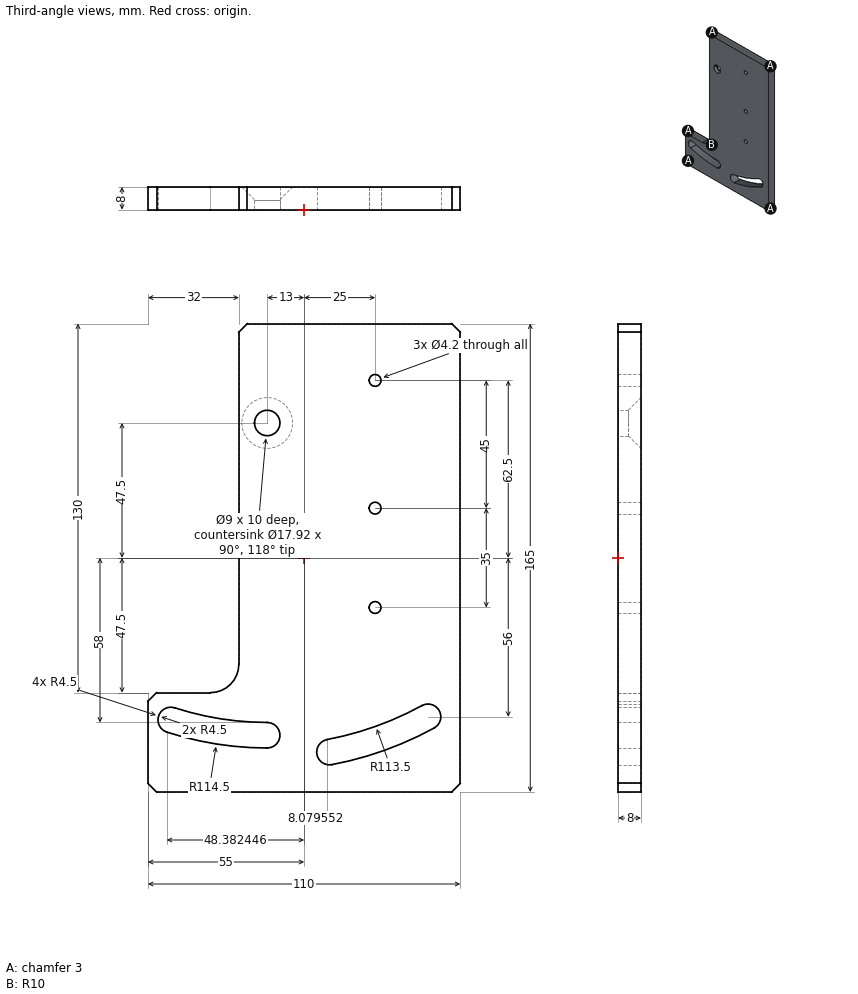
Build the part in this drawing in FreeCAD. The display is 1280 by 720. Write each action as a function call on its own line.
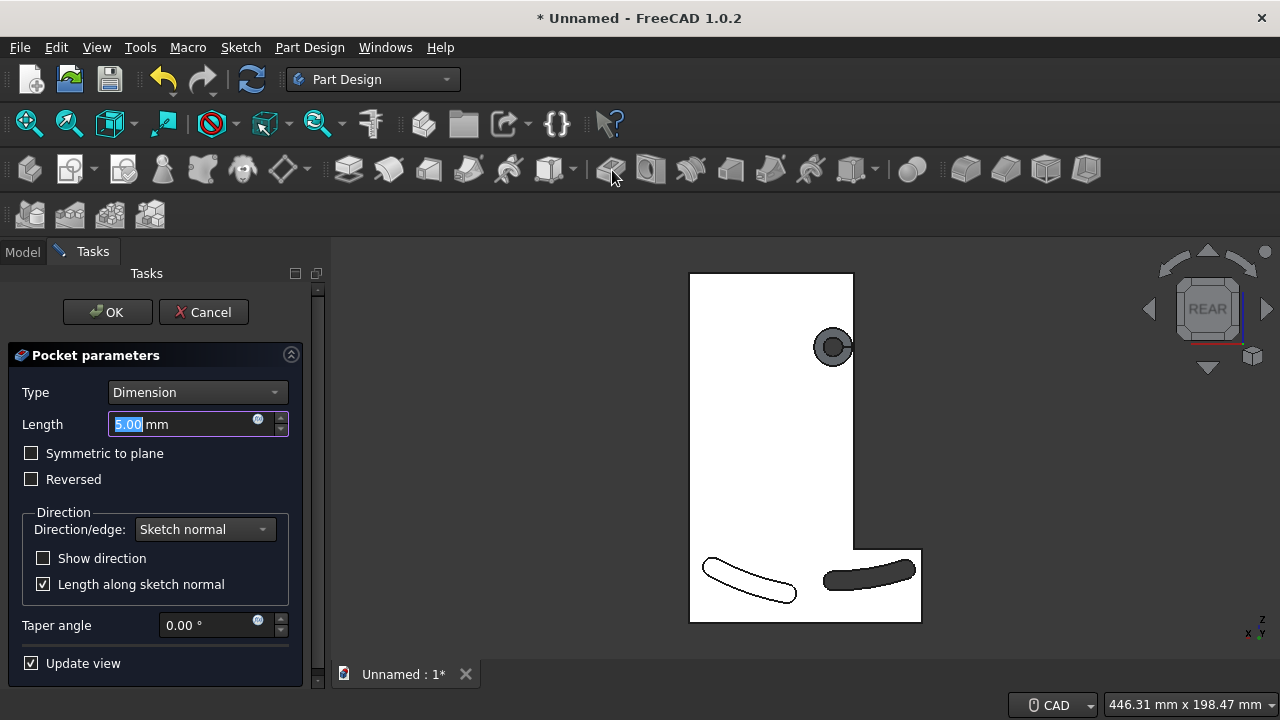
text(8)
key(Tab)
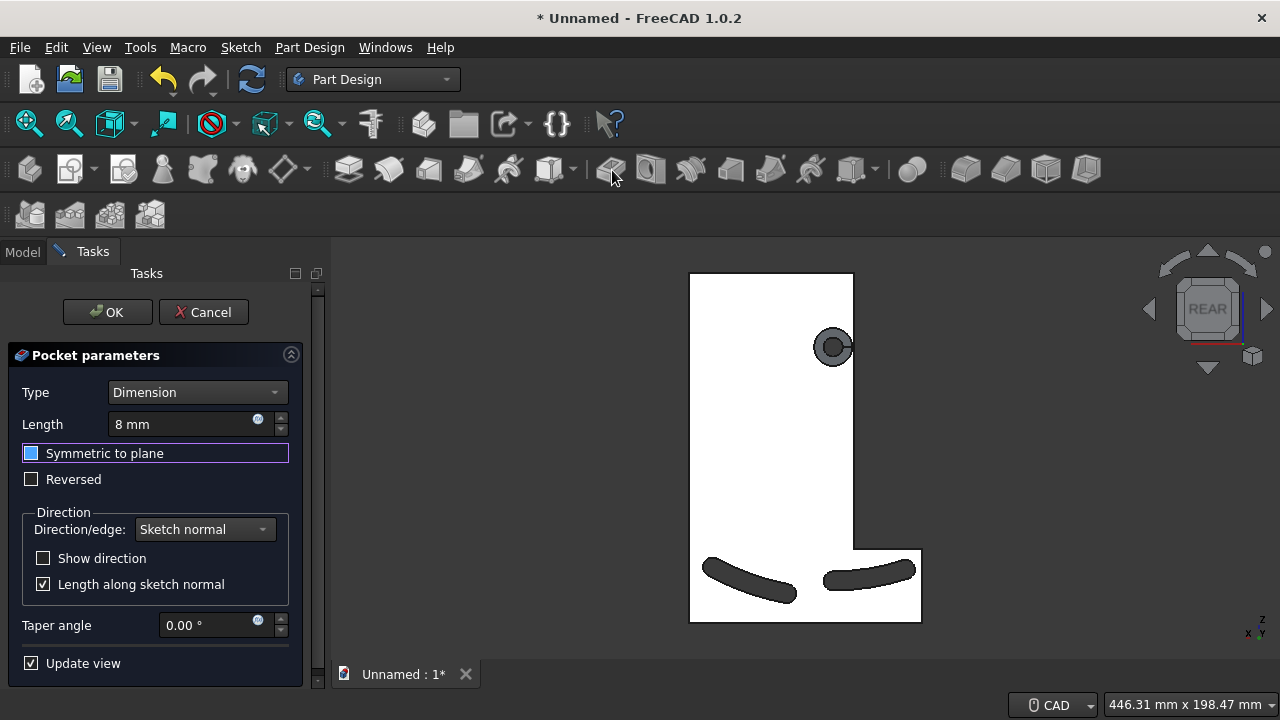
click(108, 312)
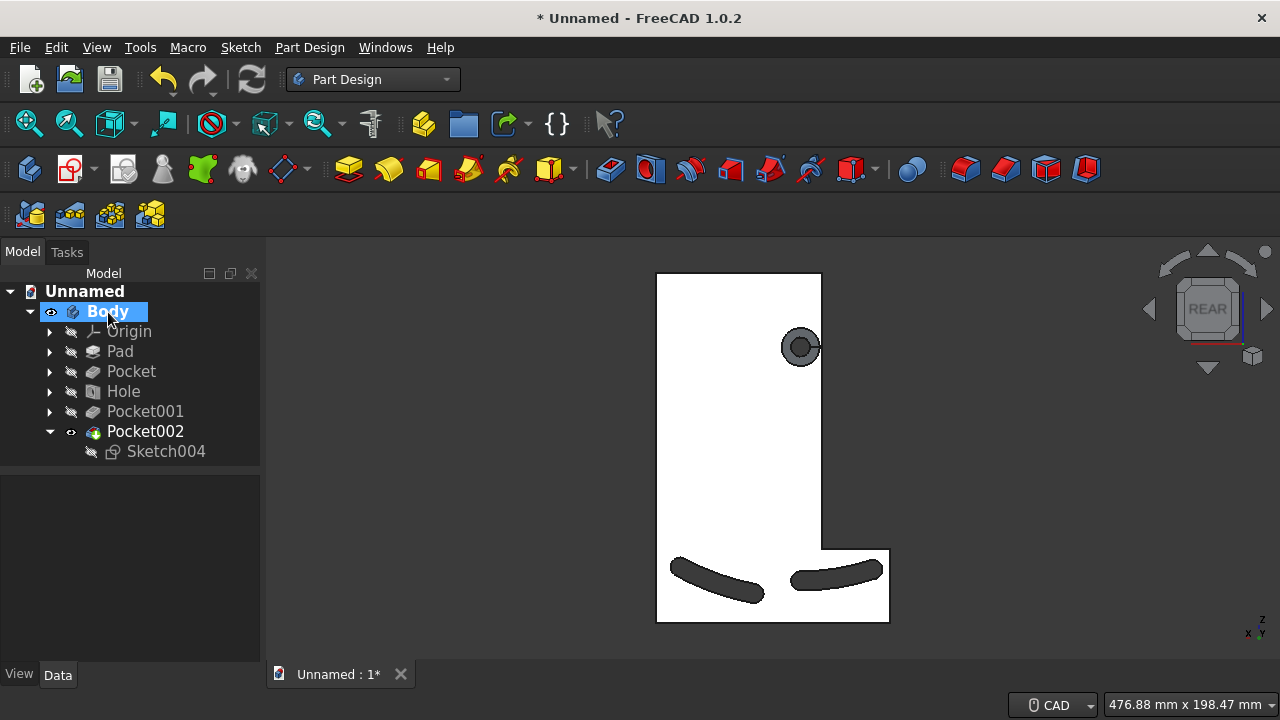
scroll(890, 548, up, 5)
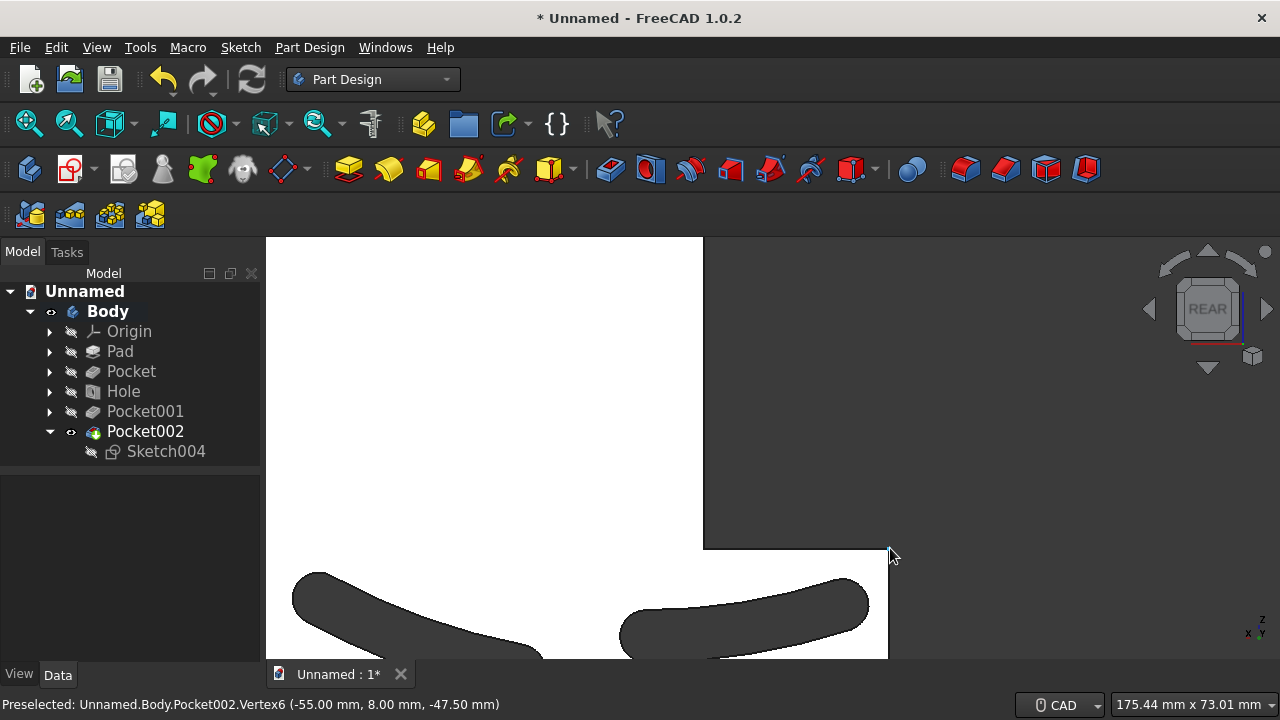
click(30, 124)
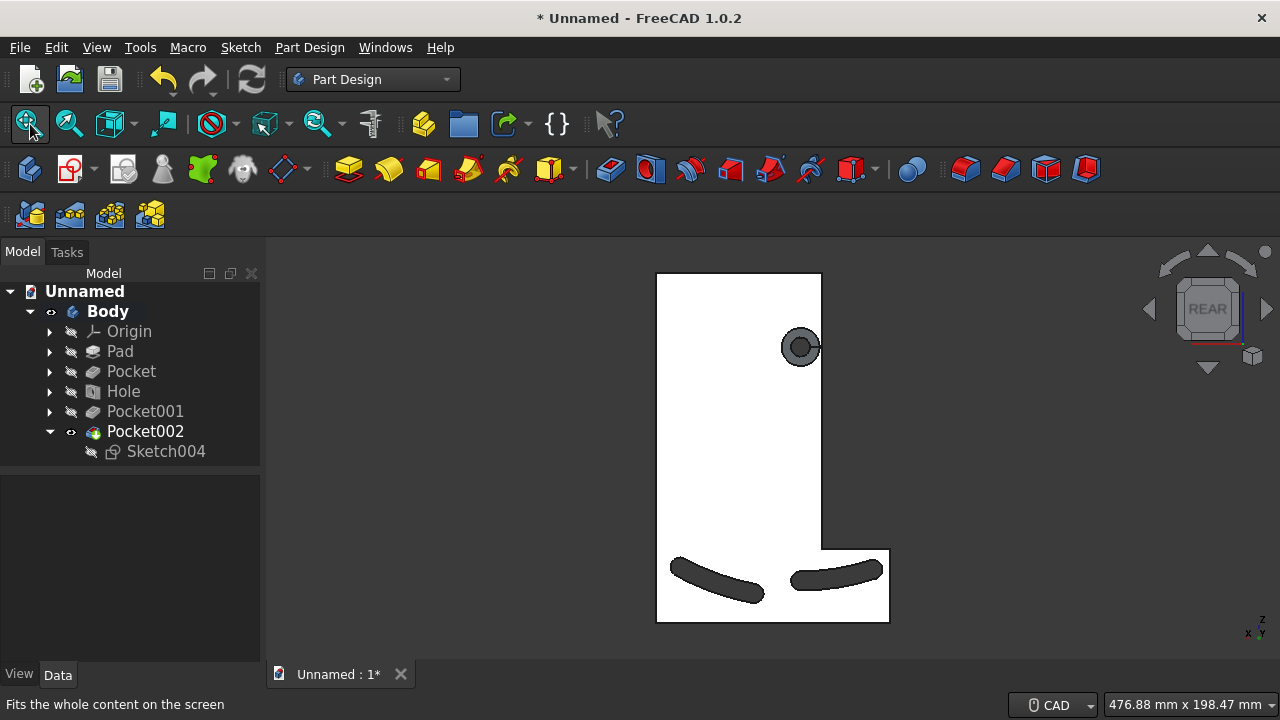
key(0)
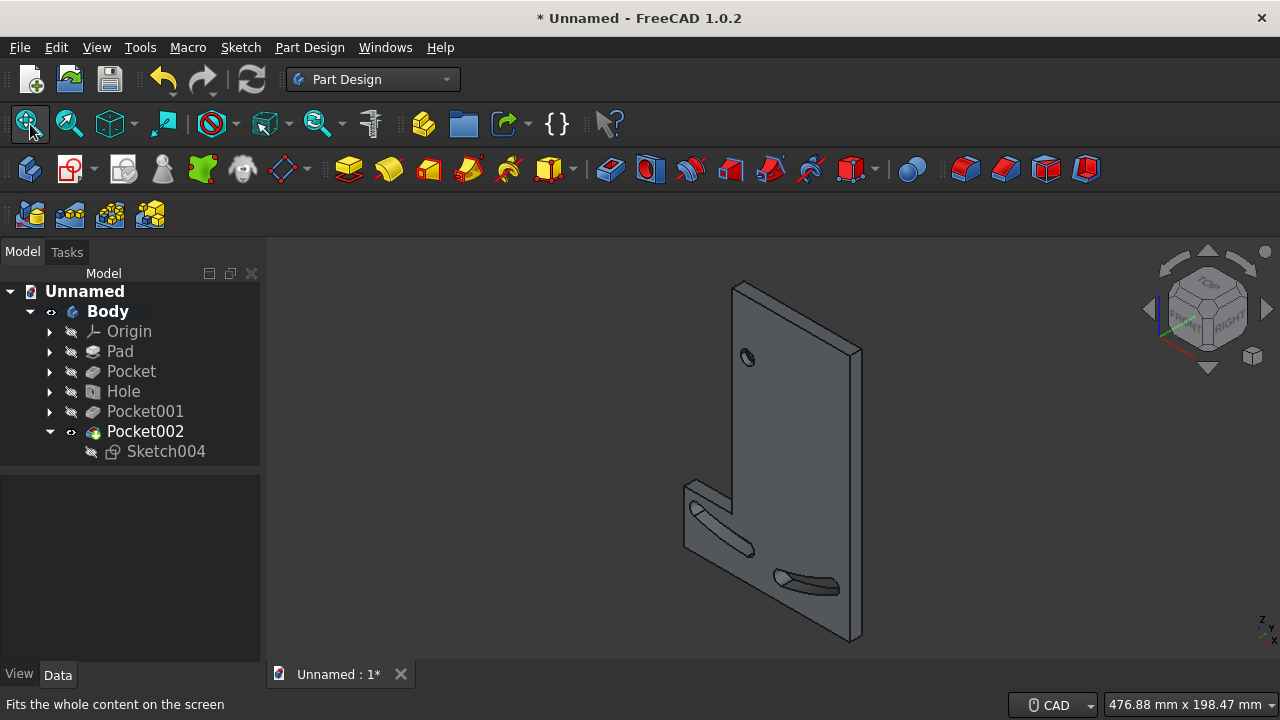
click(856, 352)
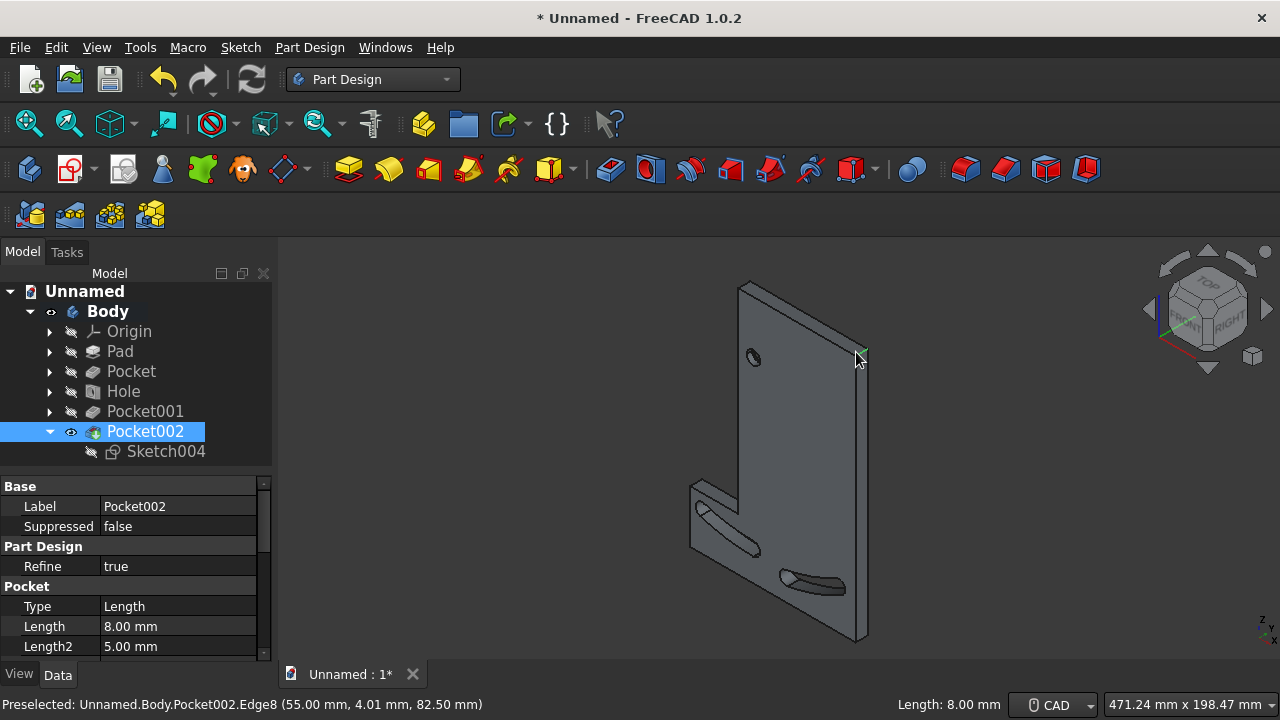
scroll(696, 482, up, 5)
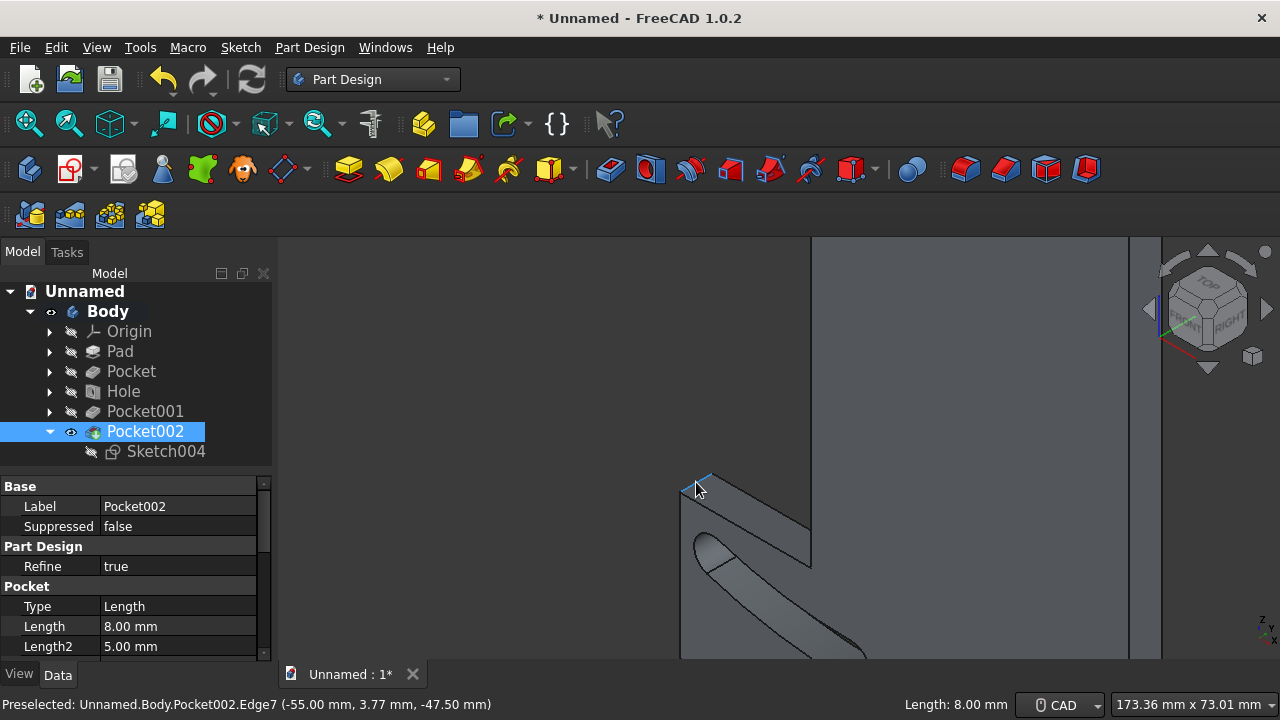
click(30, 124)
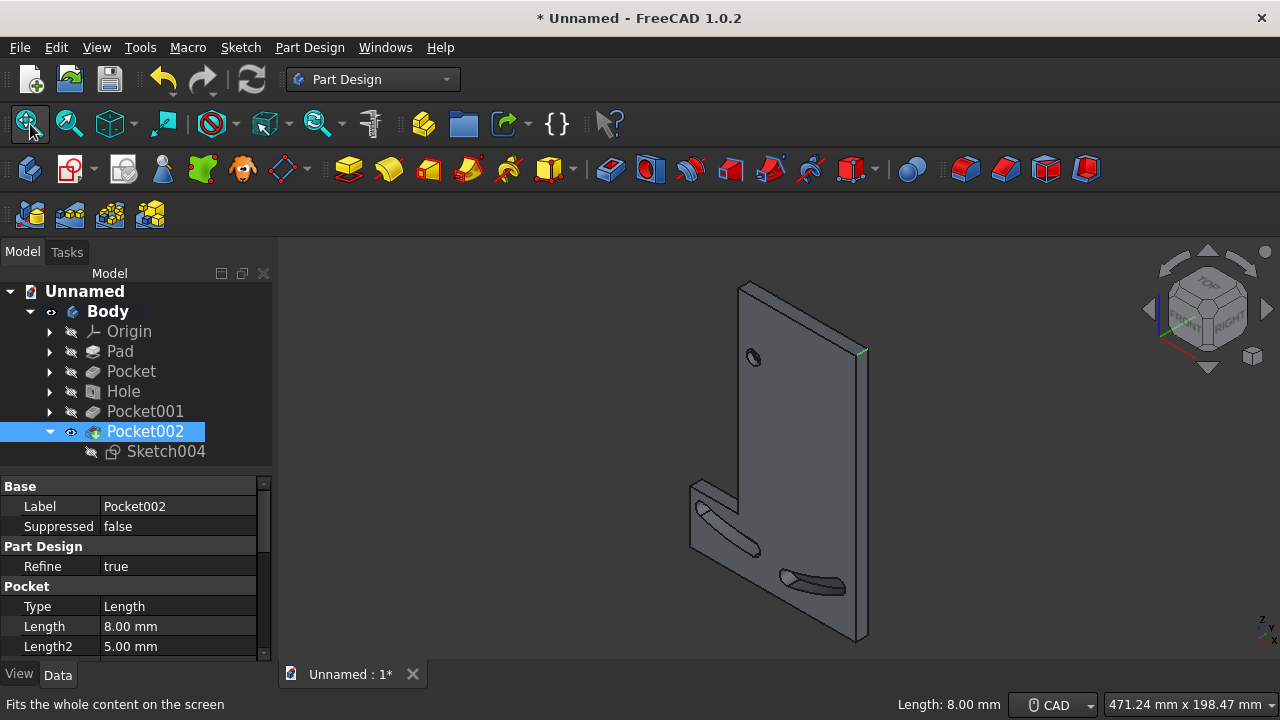
key(2)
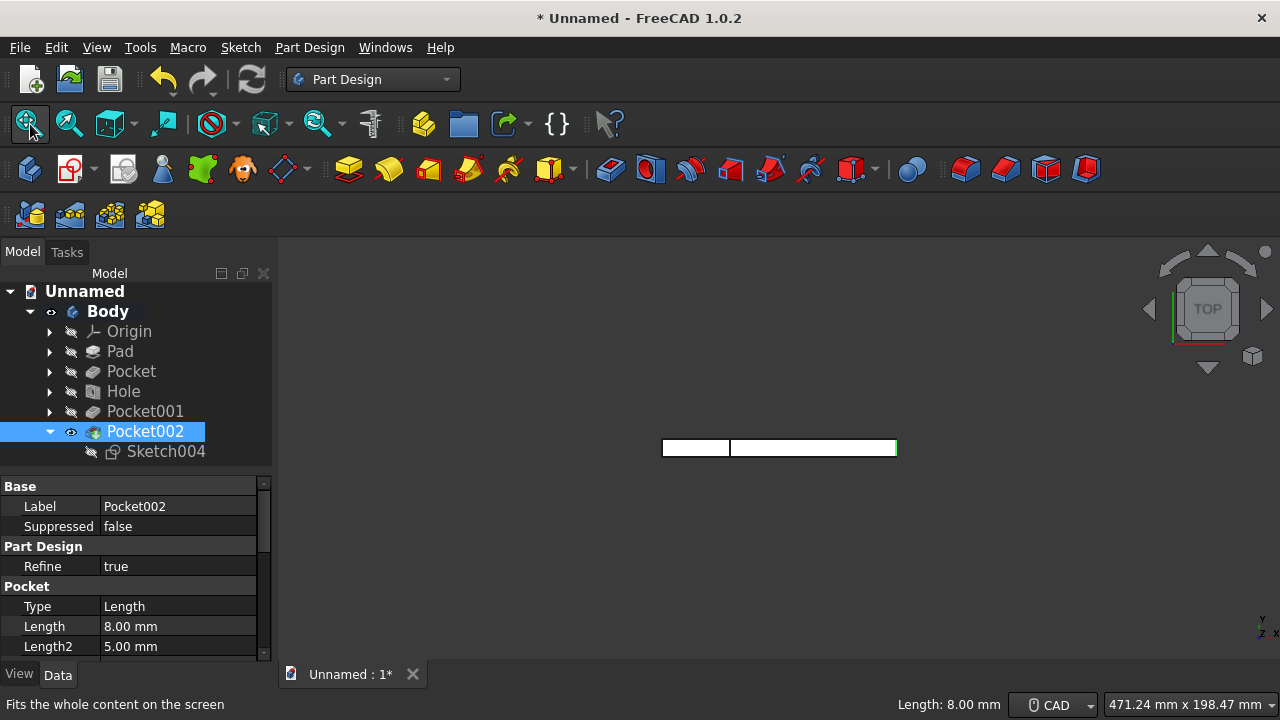
click(30, 124)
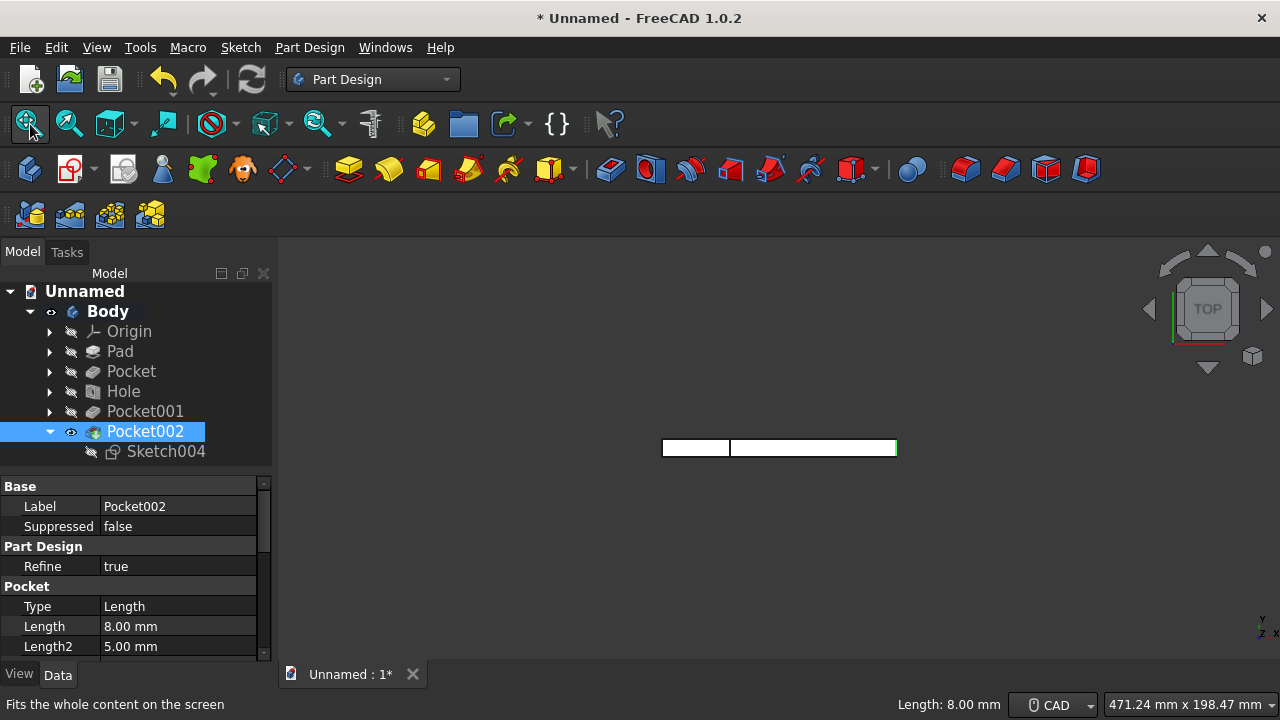
click(662, 447, ctrl)